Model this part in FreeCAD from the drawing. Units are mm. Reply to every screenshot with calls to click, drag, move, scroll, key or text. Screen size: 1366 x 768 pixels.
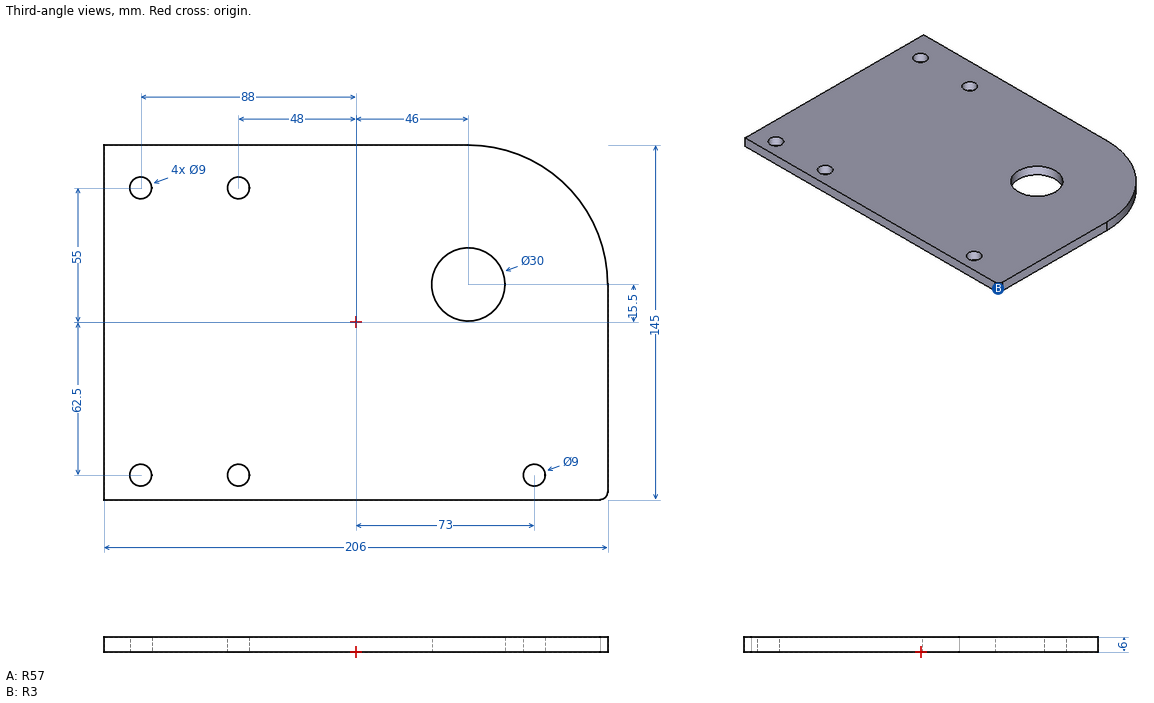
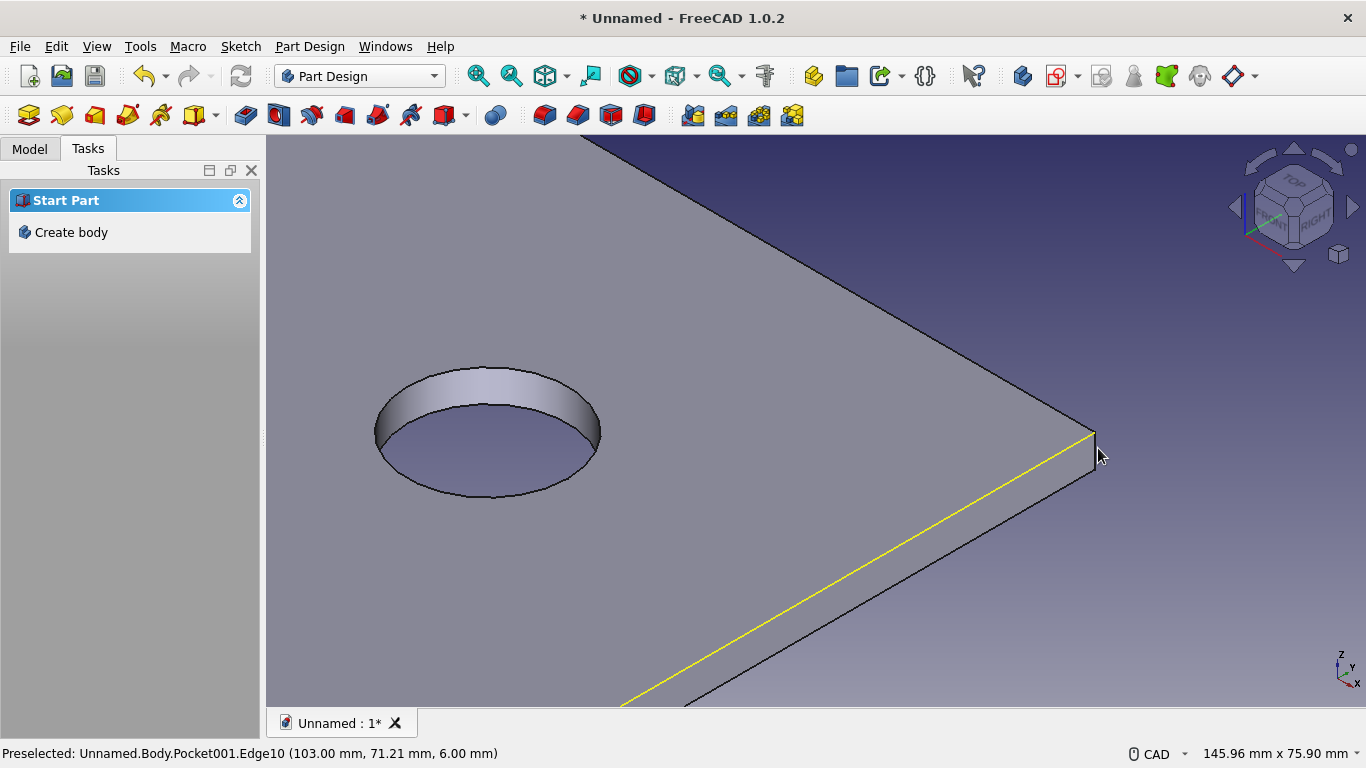
click(479, 76)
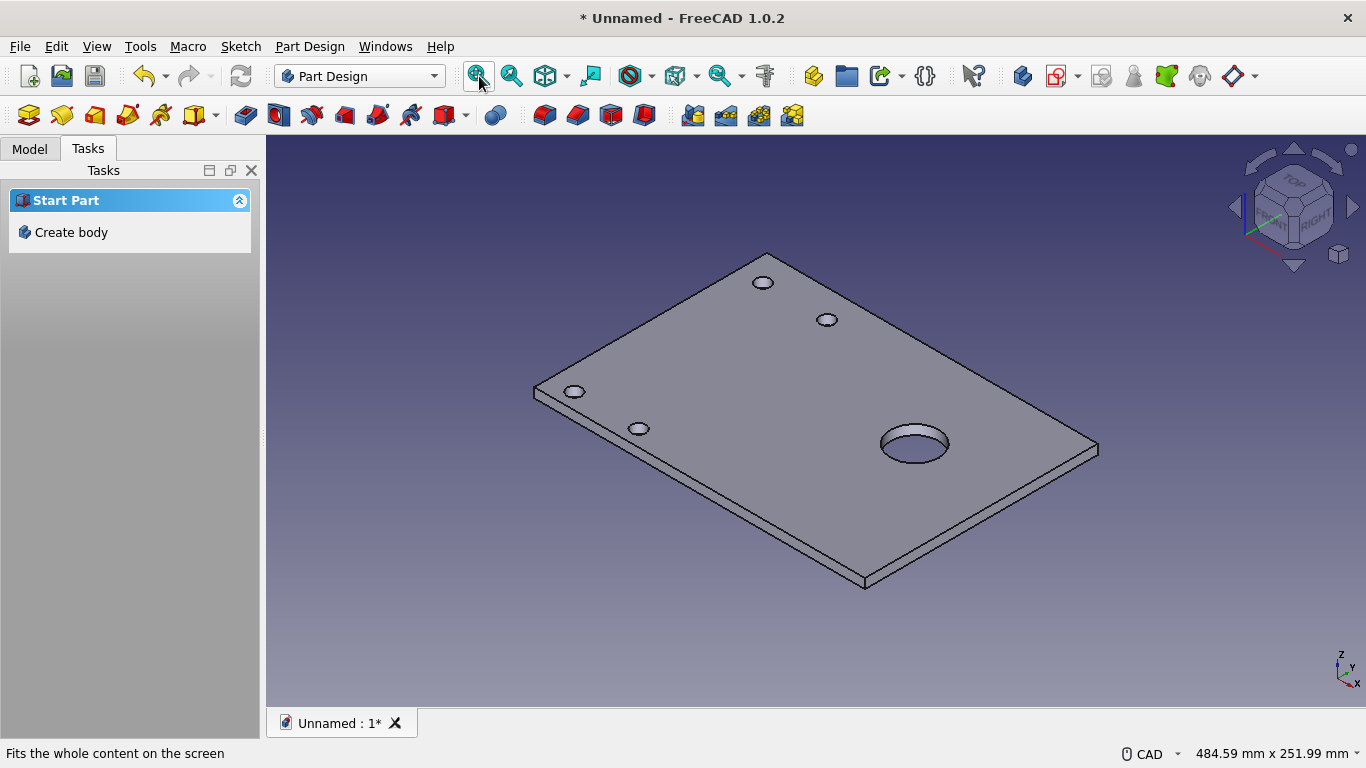
key(2)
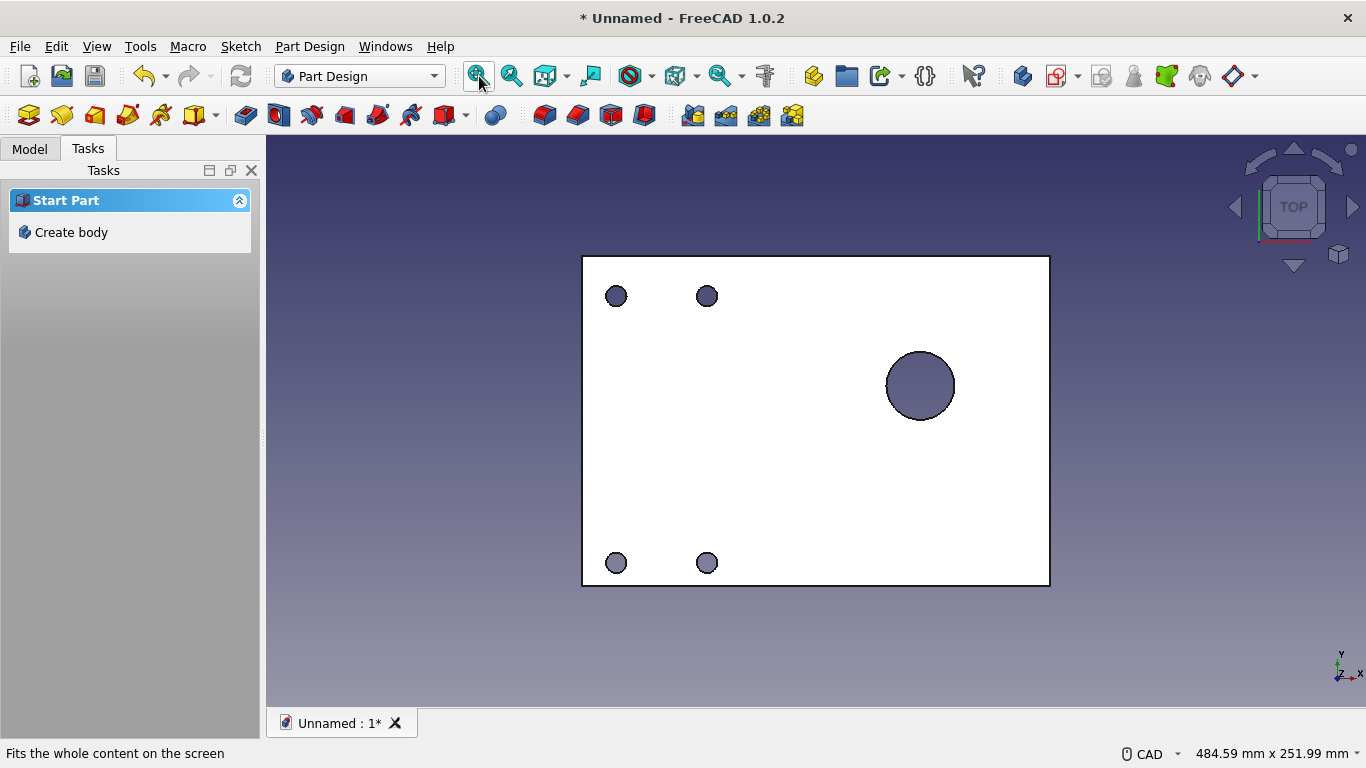
scroll(1050, 255, up, 6)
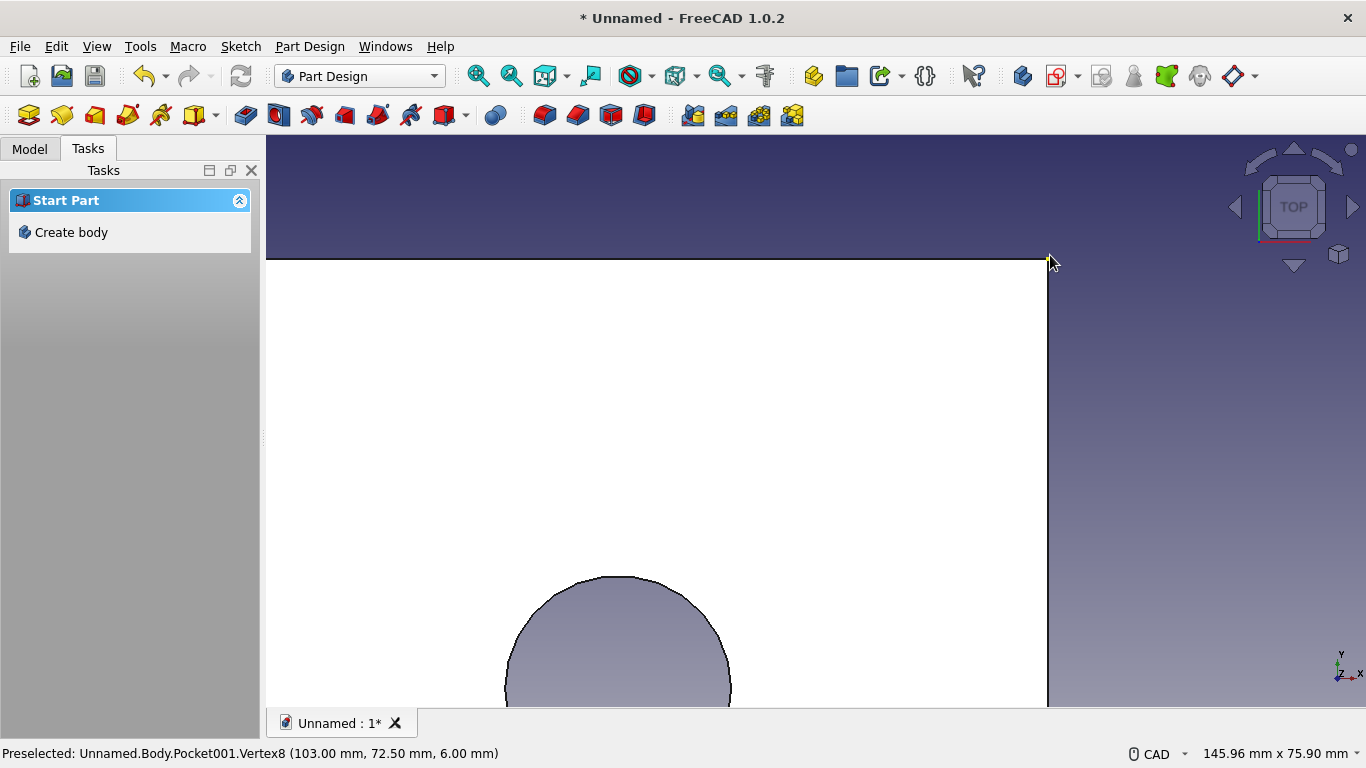
click(479, 76)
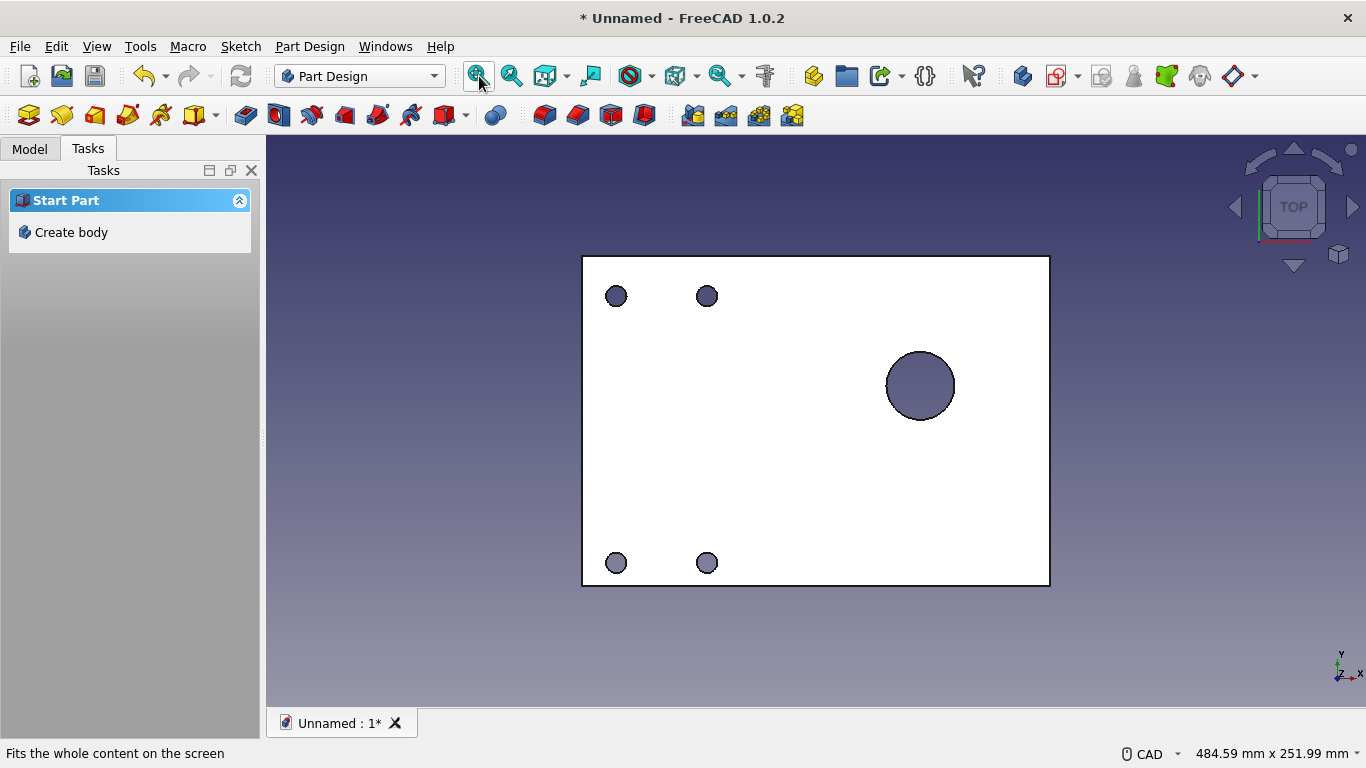
key(1)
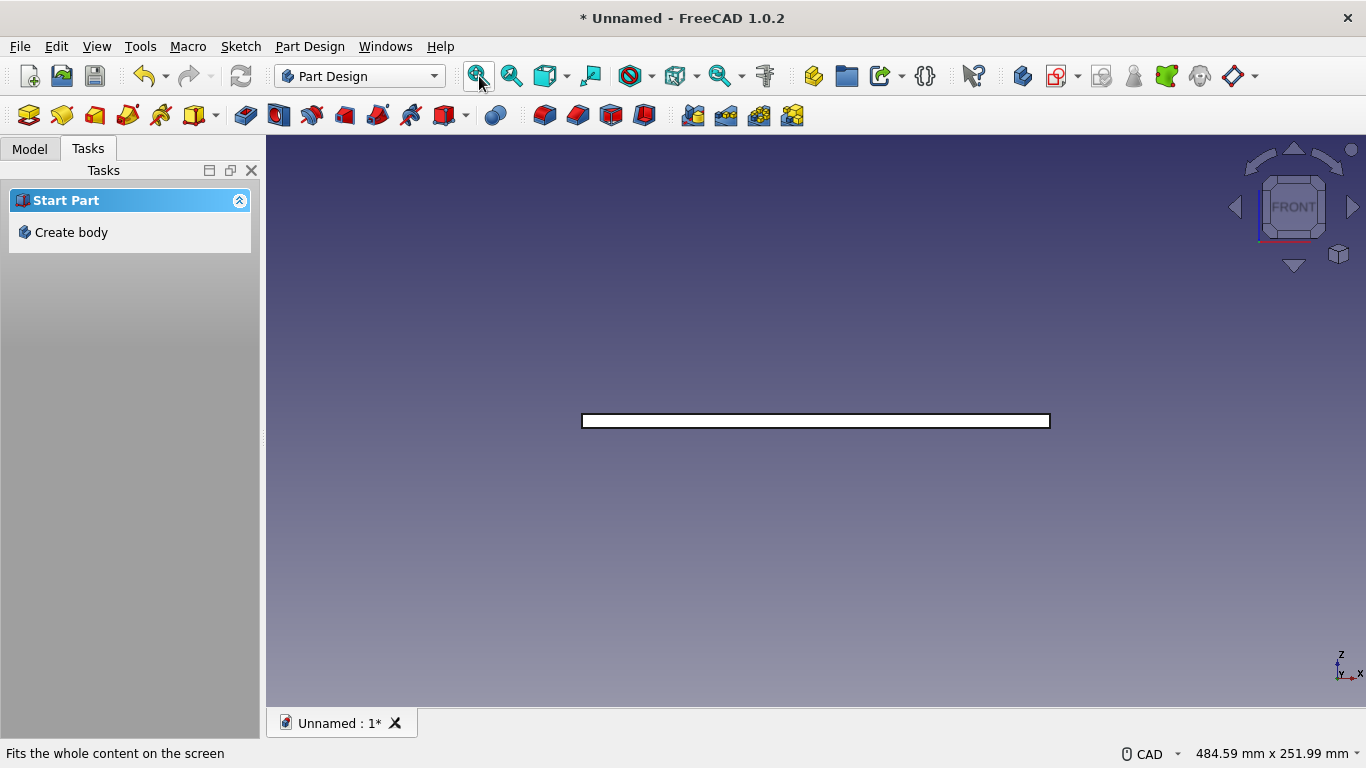
click(479, 76)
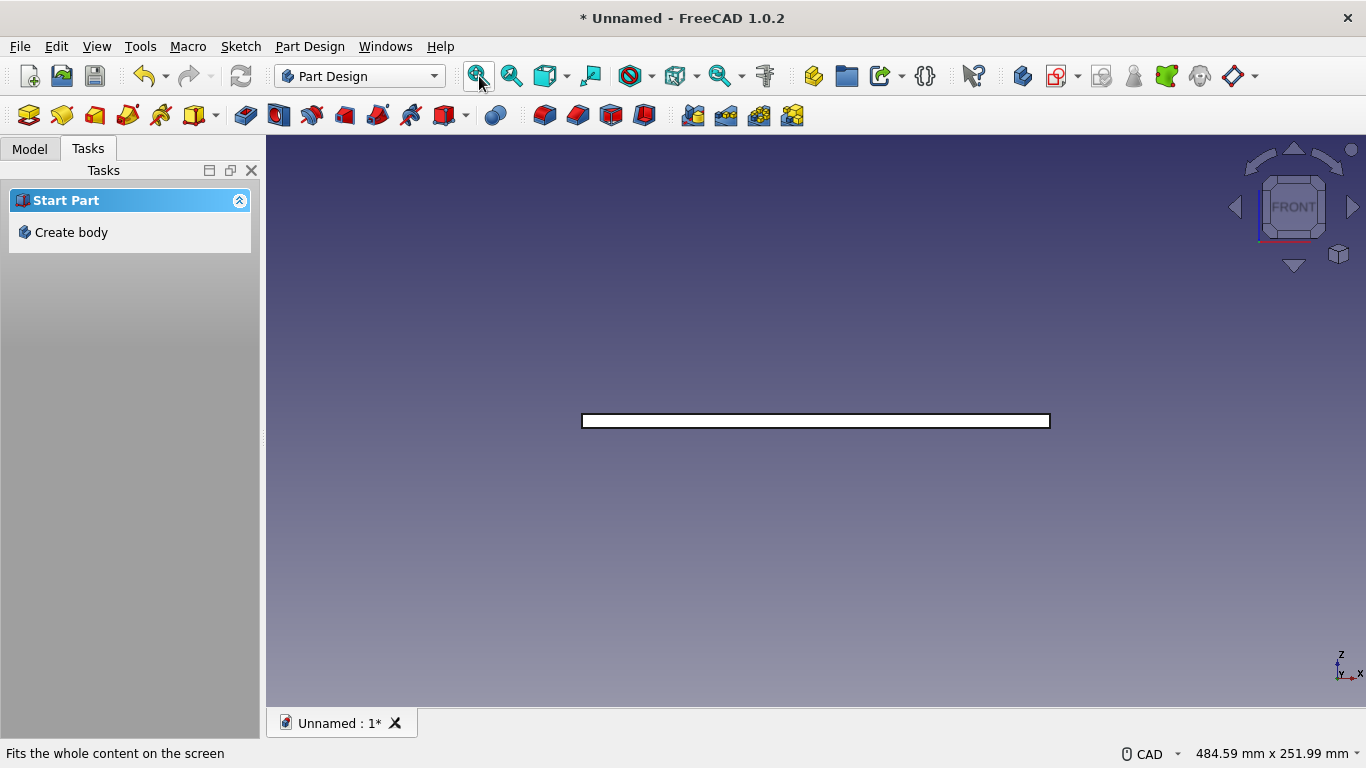
scroll(1050, 420, up, 6)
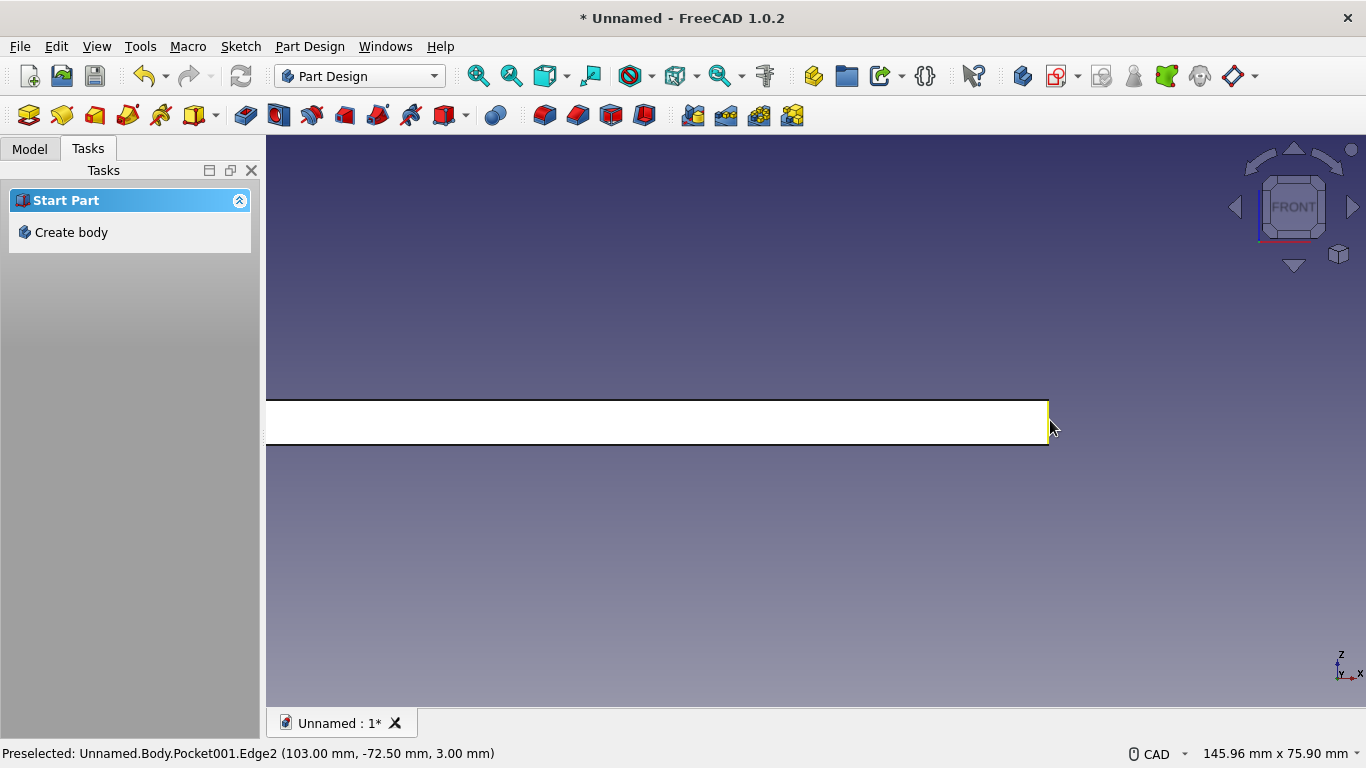
click(479, 76)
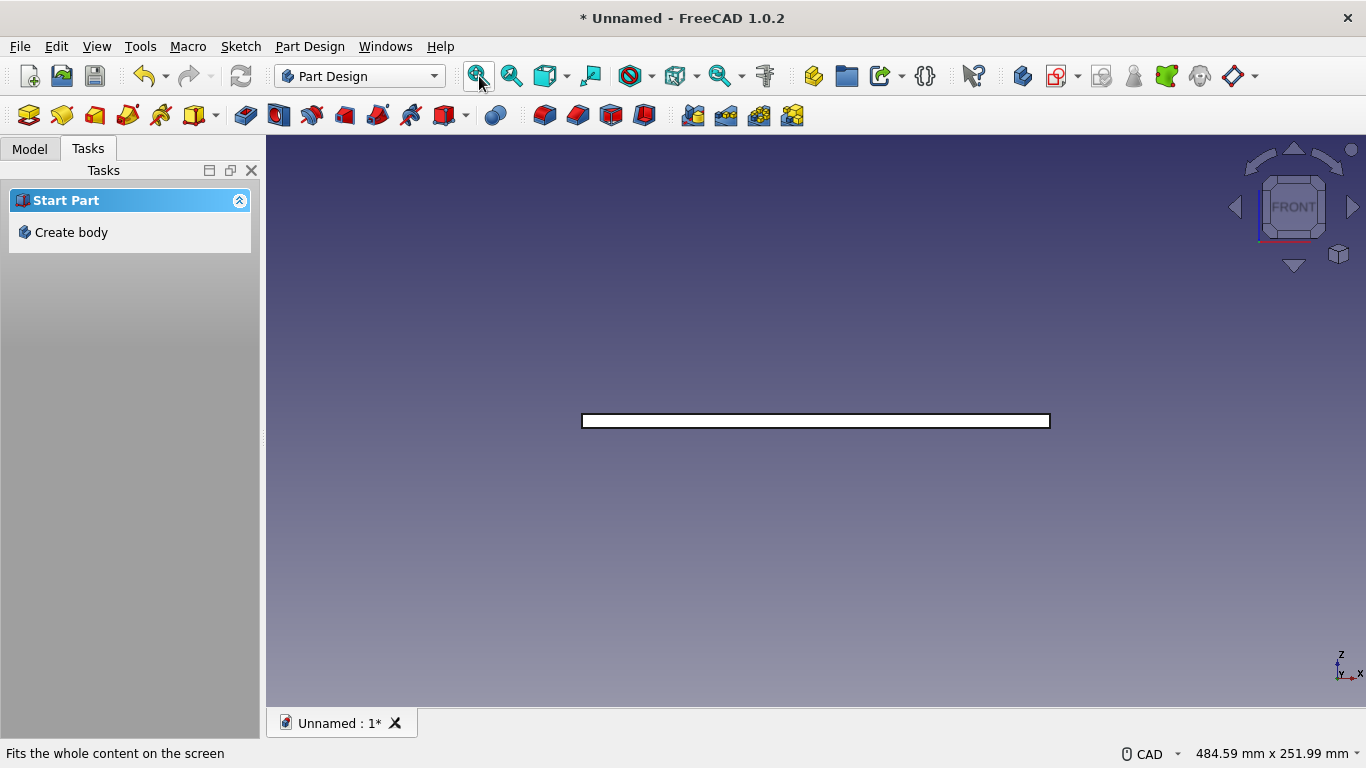
key(3)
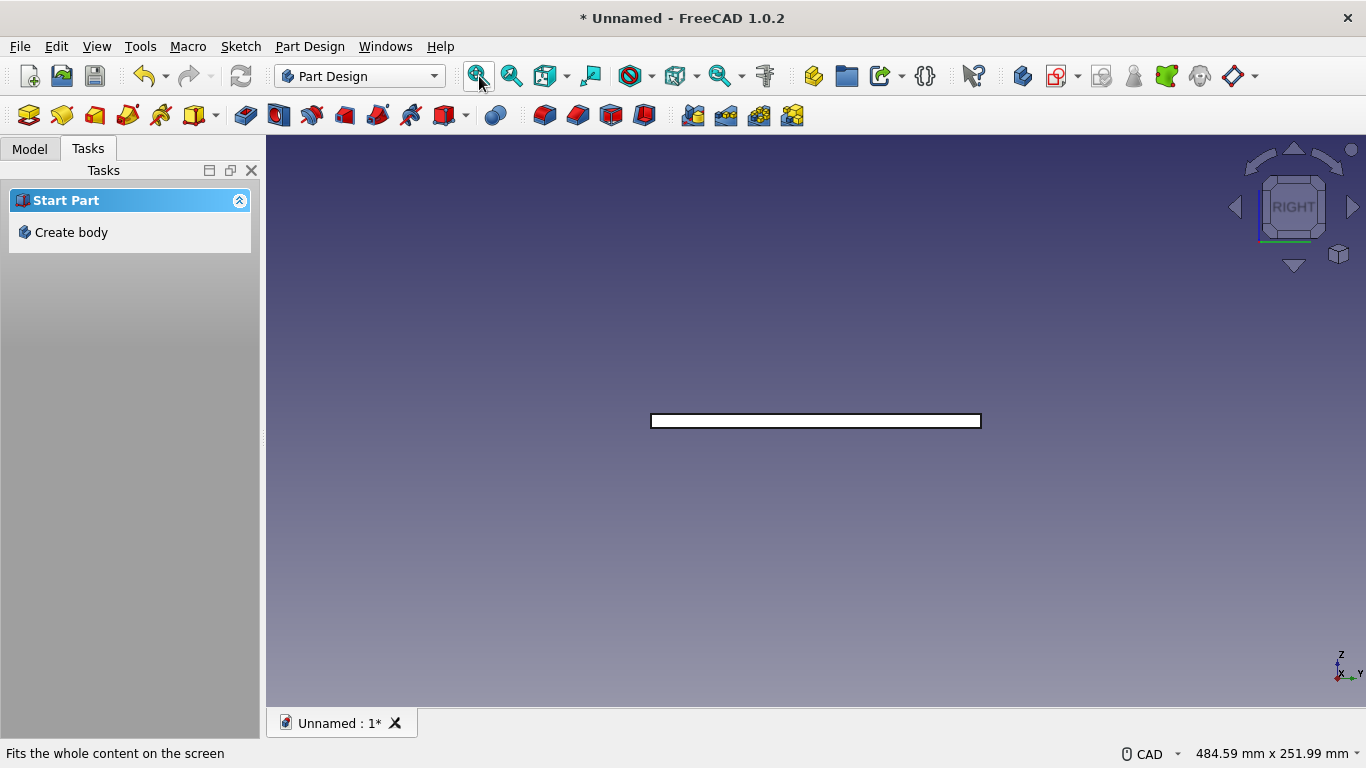
click(479, 76)